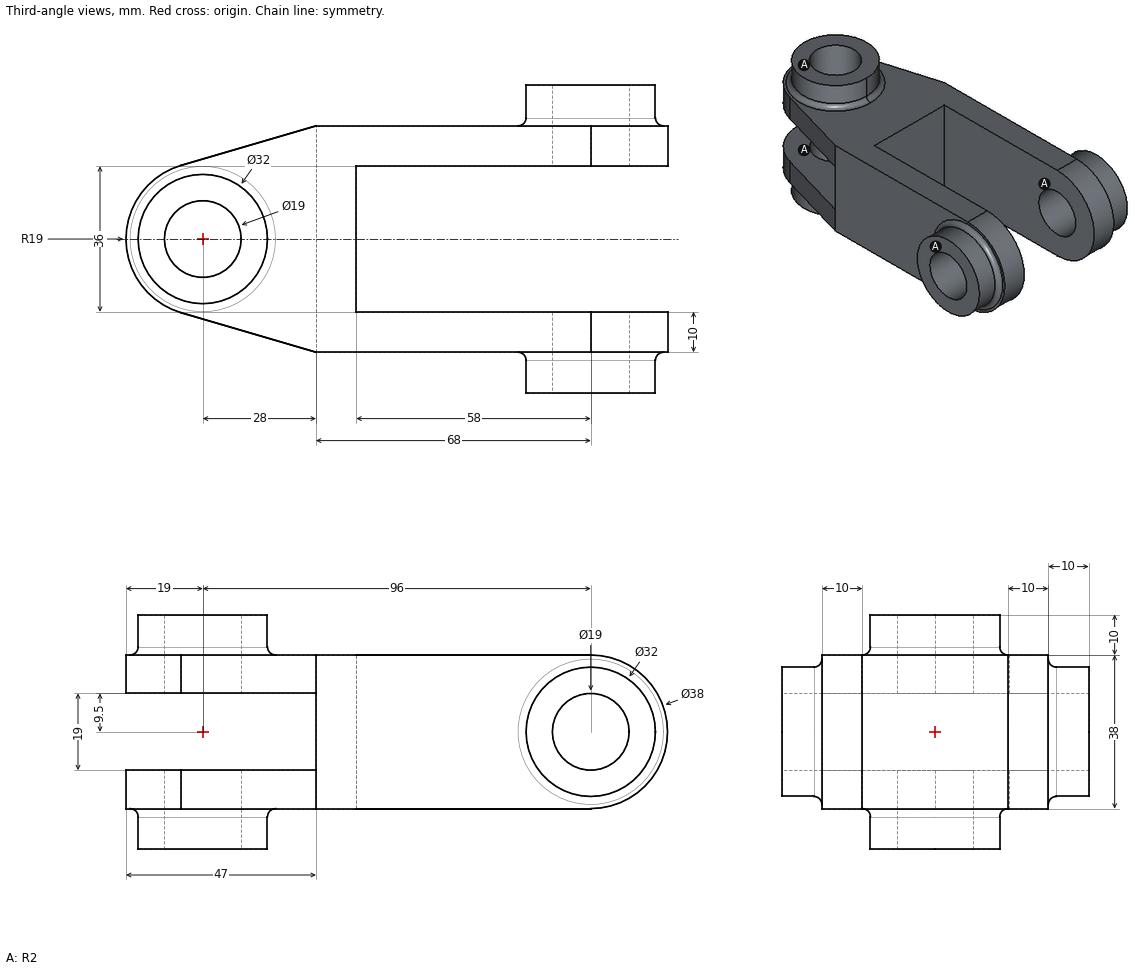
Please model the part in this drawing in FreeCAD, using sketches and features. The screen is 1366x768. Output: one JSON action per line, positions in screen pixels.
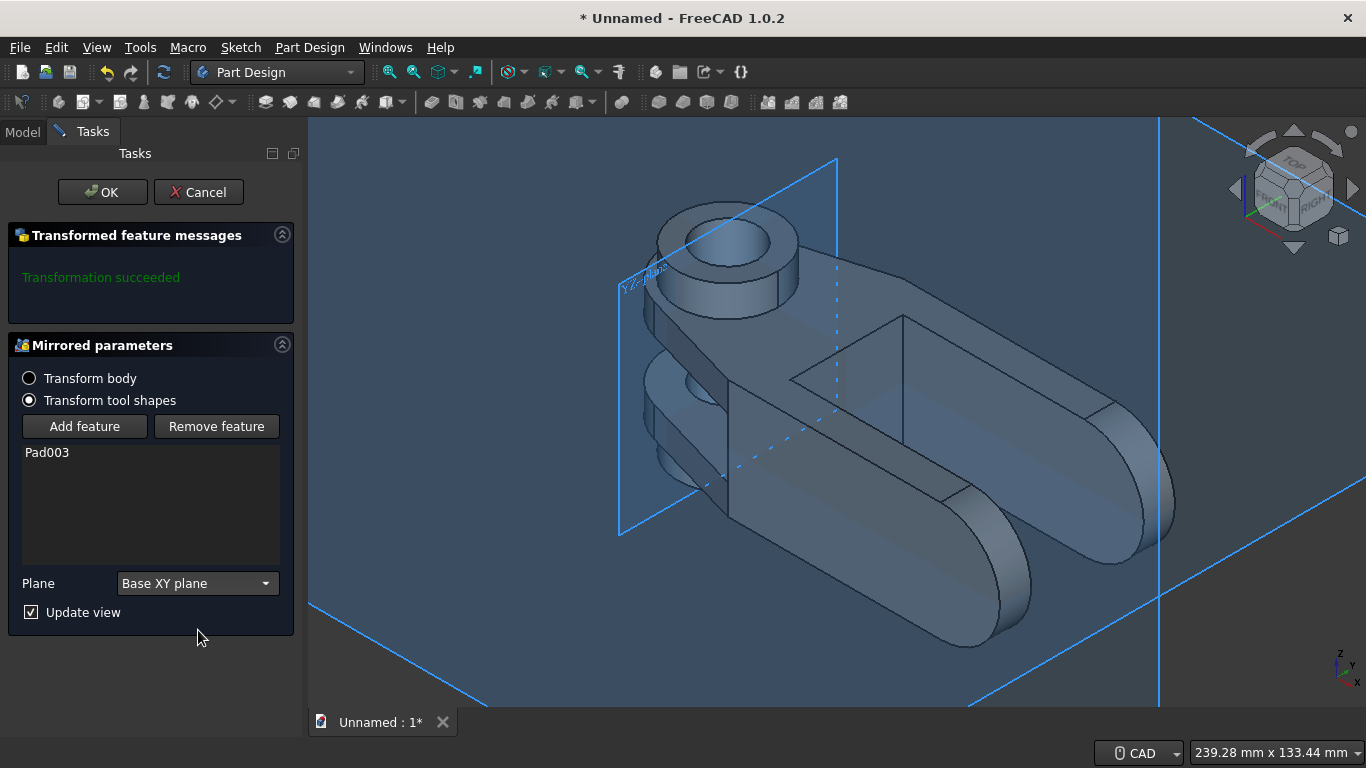
{"action": "left_click", "coordinate": [103, 192]}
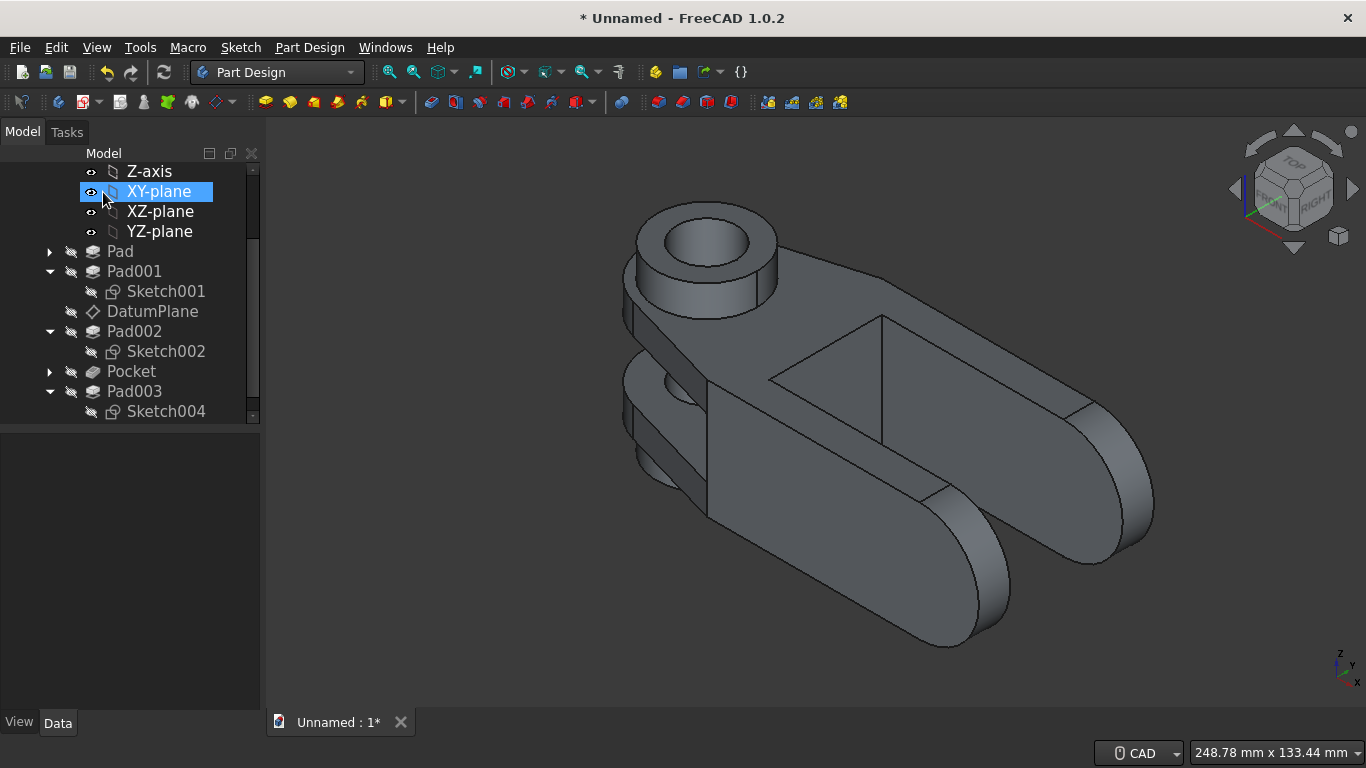
{"action": "left_click", "coordinate": [390, 72]}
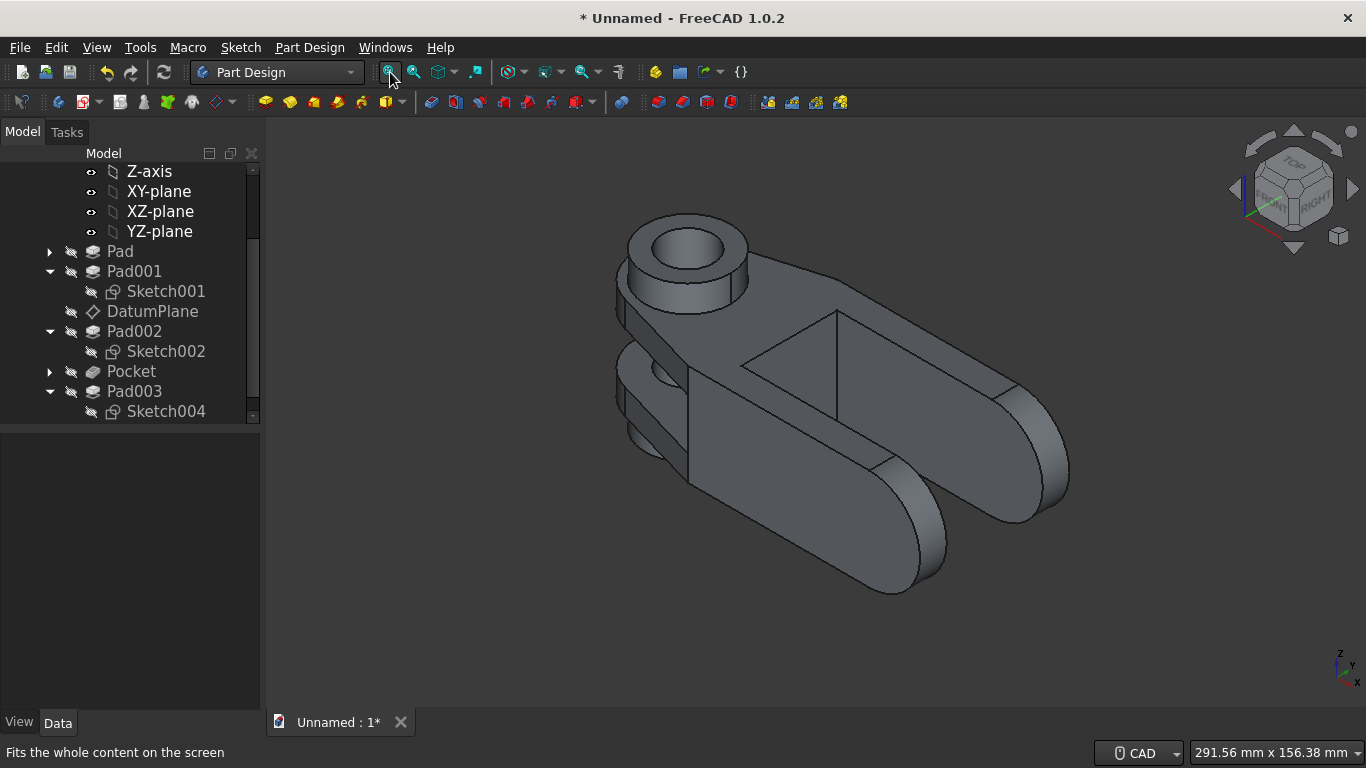
{"action": "key", "text": "4"}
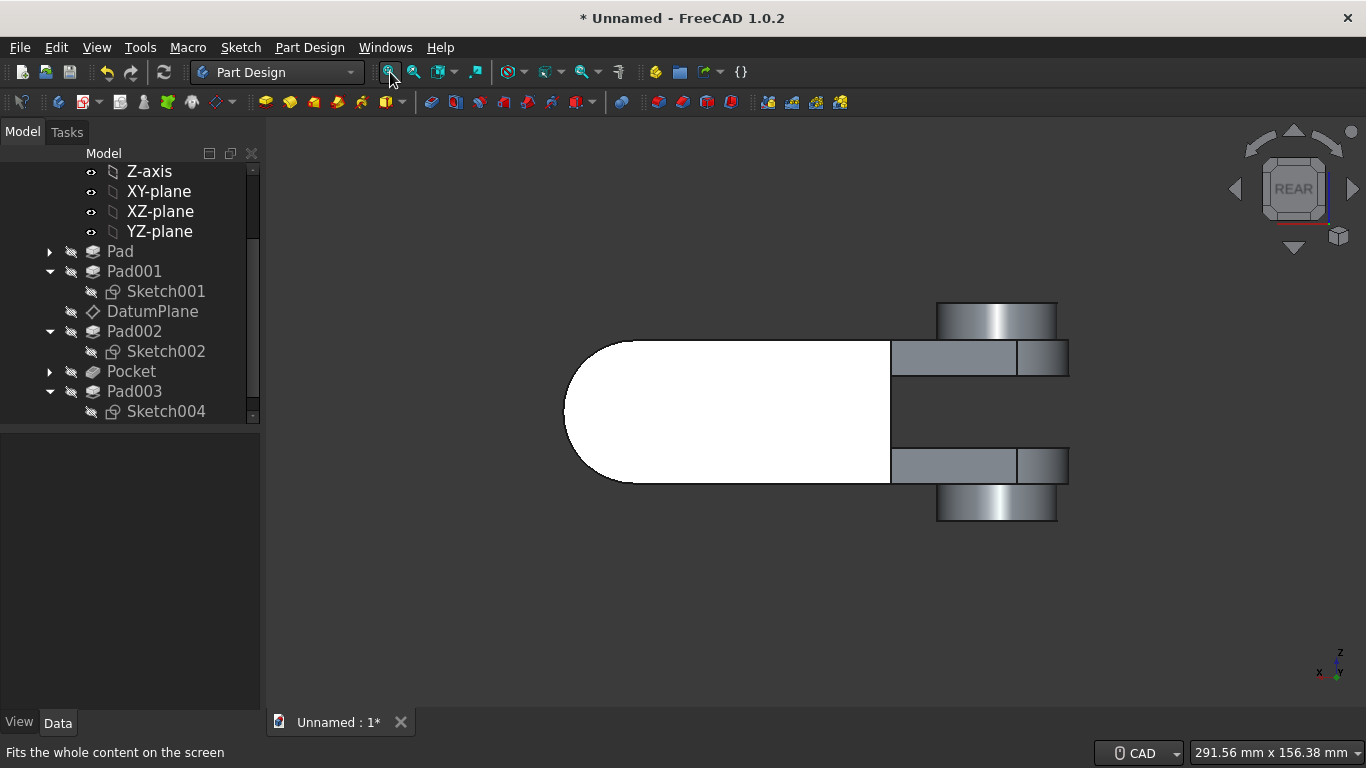
{"action": "left_click", "coordinate": [680, 411]}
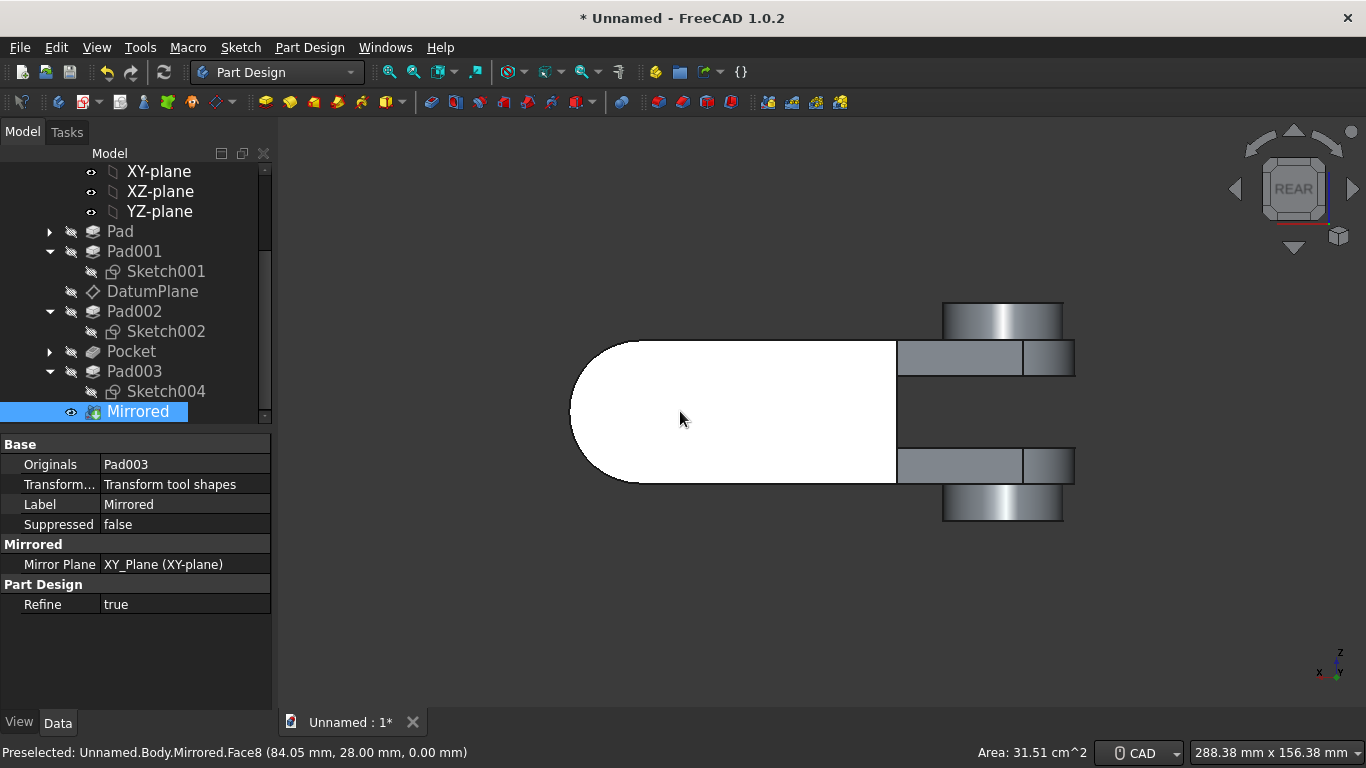
{"action": "left_click", "coordinate": [84, 102]}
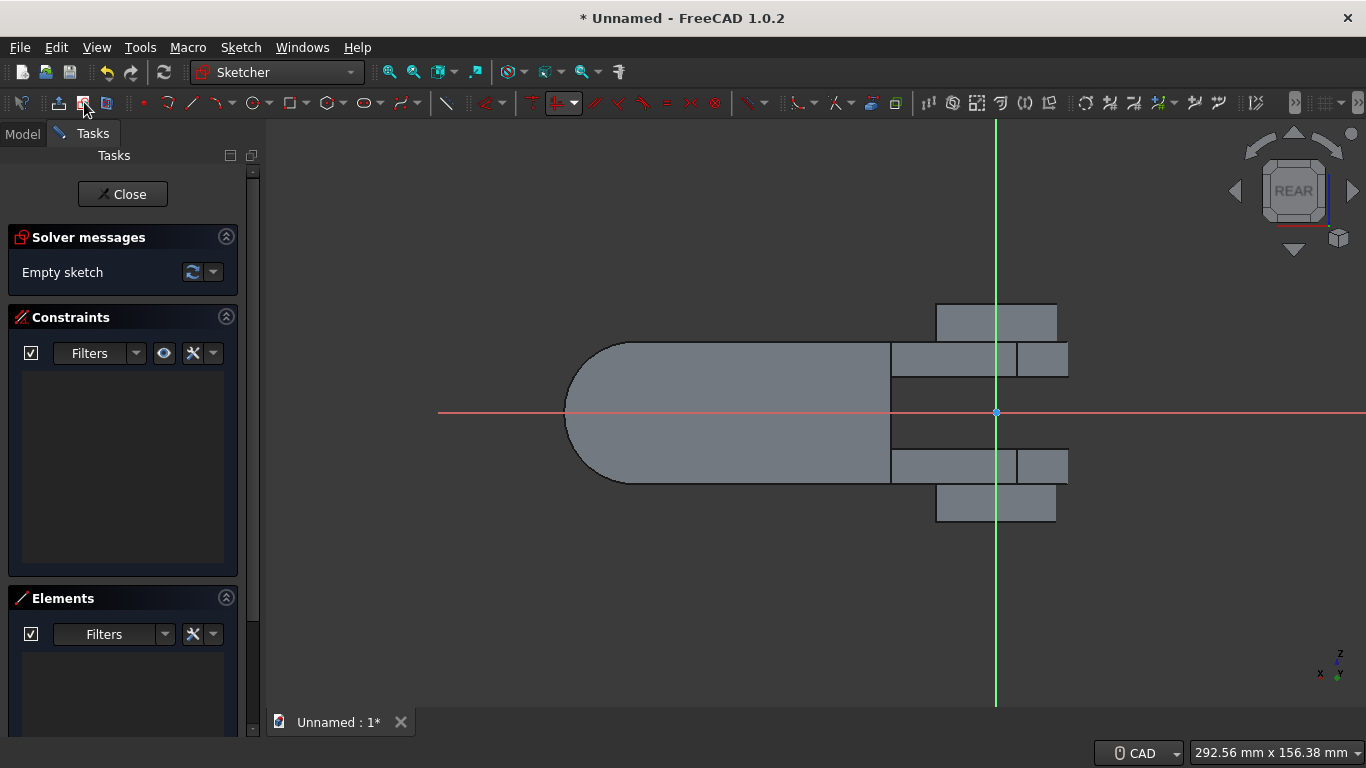
{"action": "scroll", "coordinate": [587, 413], "scroll_direction": "up", "scroll_amount": 6}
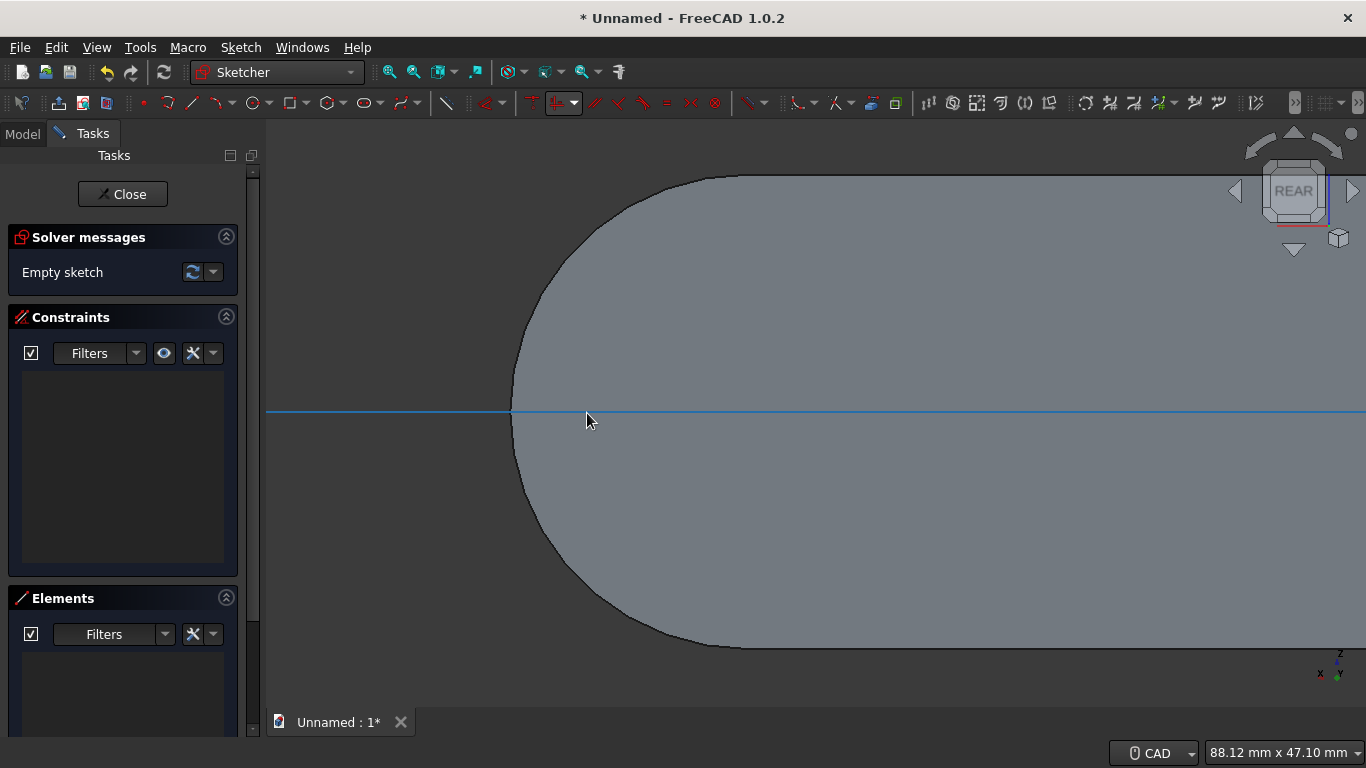
{"action": "left_click", "coordinate": [254, 104]}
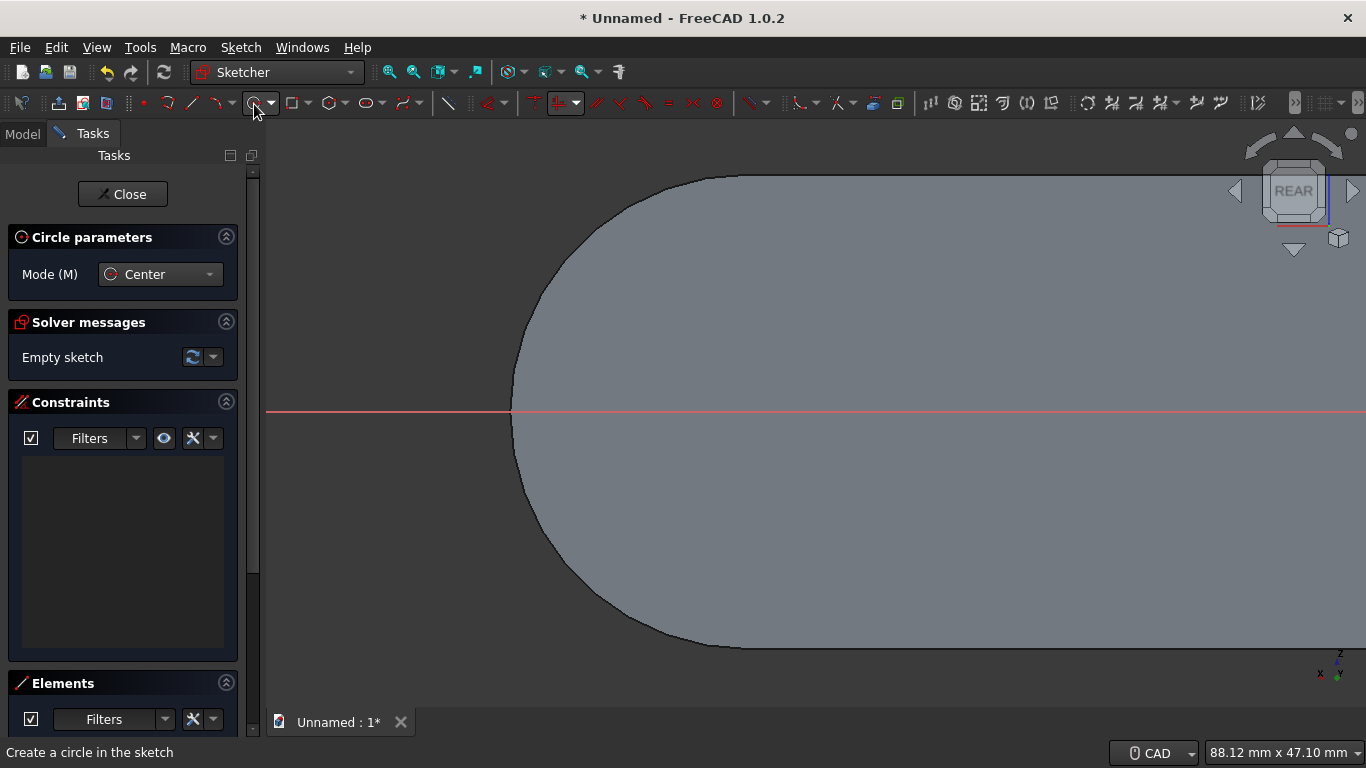
{"action": "left_click", "coordinate": [747, 412]}
{"action": "left_click", "coordinate": [889, 271]}
{"action": "key", "text": "Escape"}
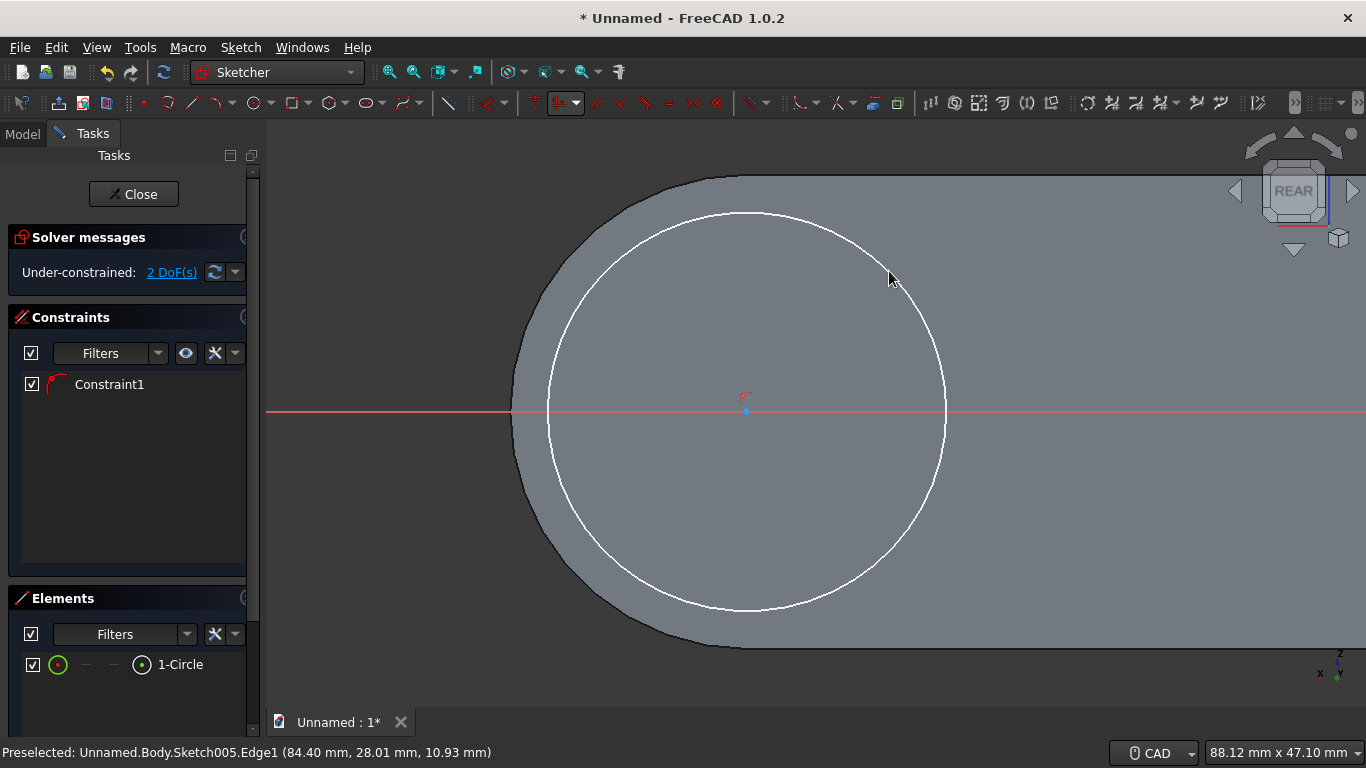
{"action": "key", "text": "d"}